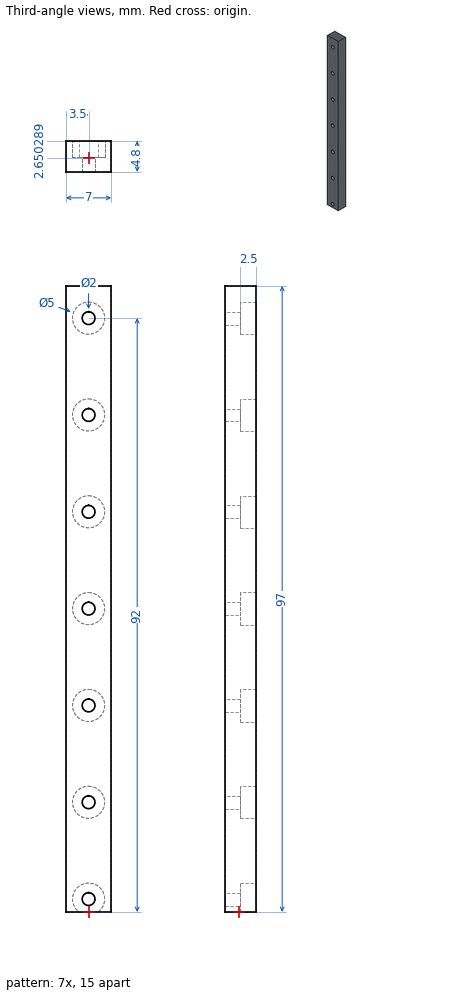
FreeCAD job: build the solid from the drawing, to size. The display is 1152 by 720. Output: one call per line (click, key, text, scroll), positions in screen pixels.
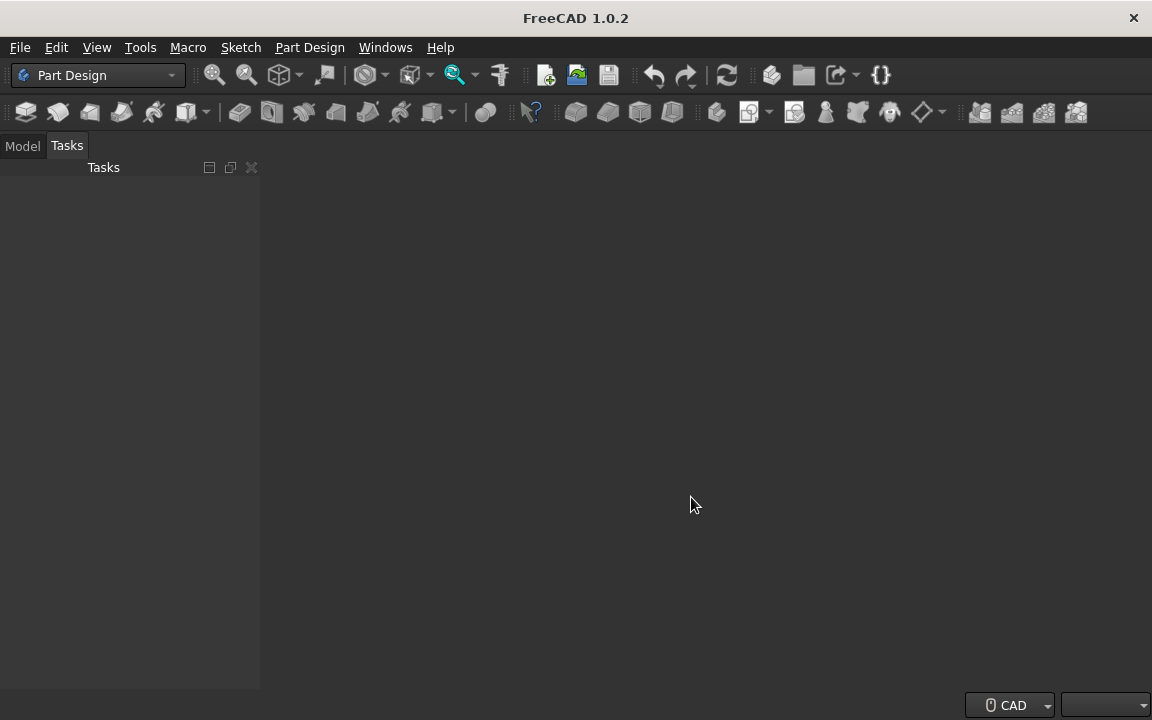
click(546, 76)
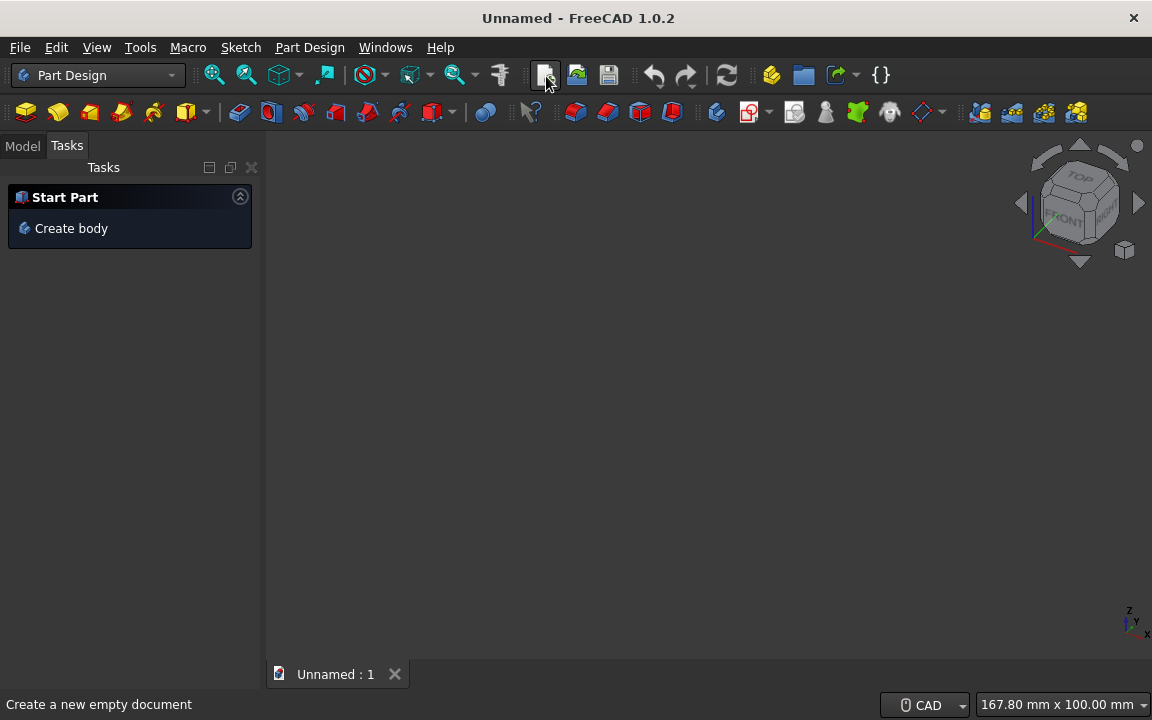
click(750, 112)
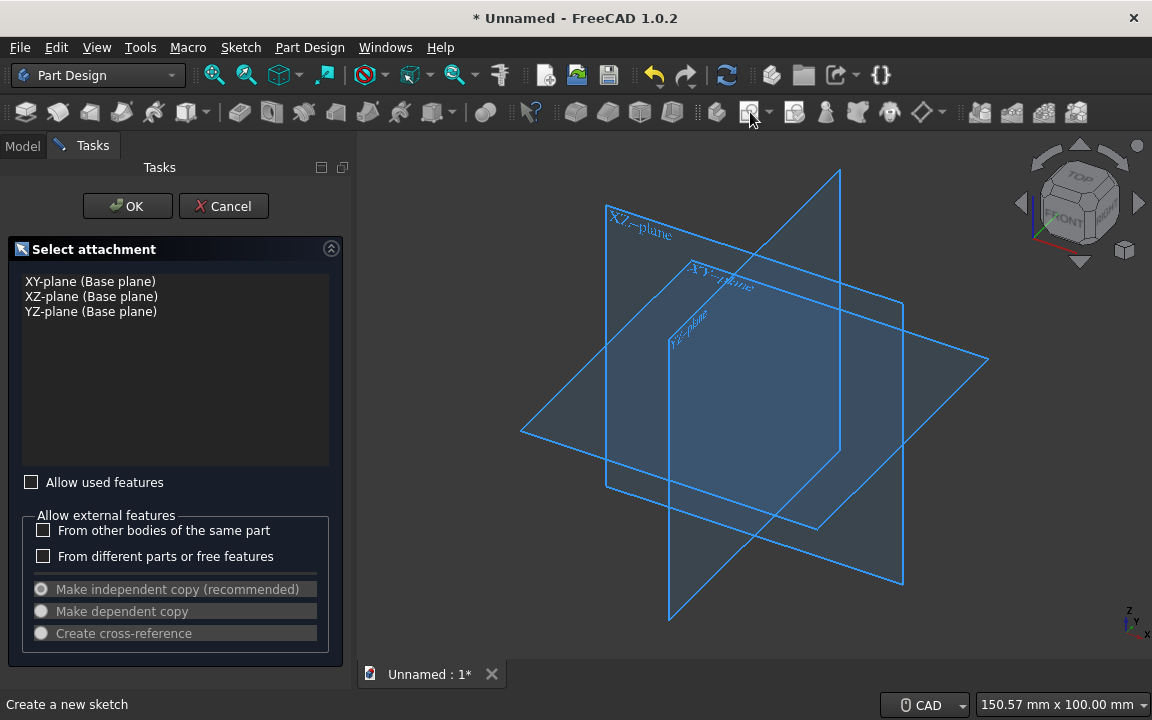
click(82, 282)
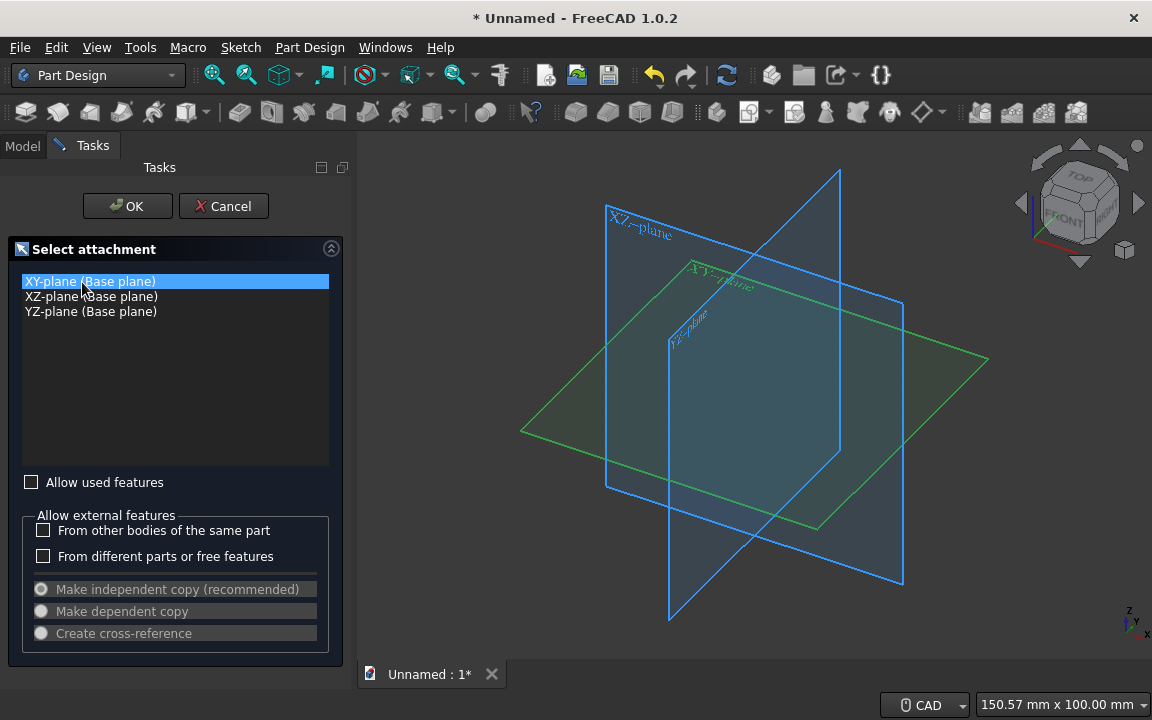
click(128, 206)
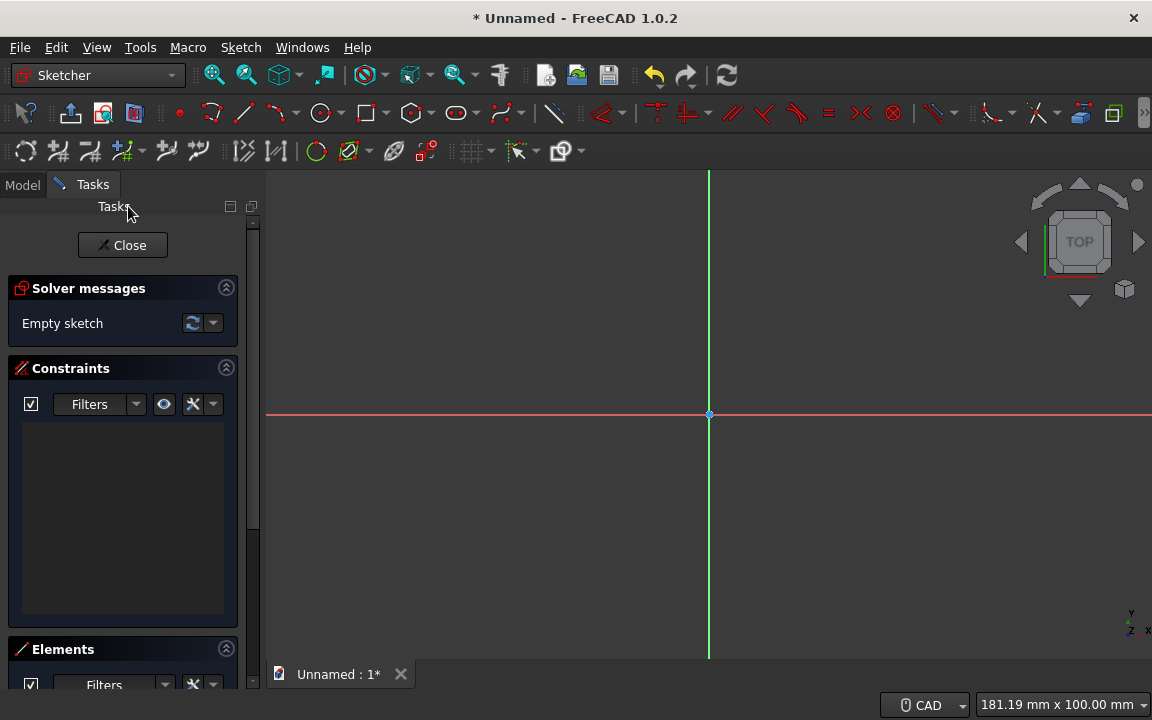
scroll(714, 413, up, 13)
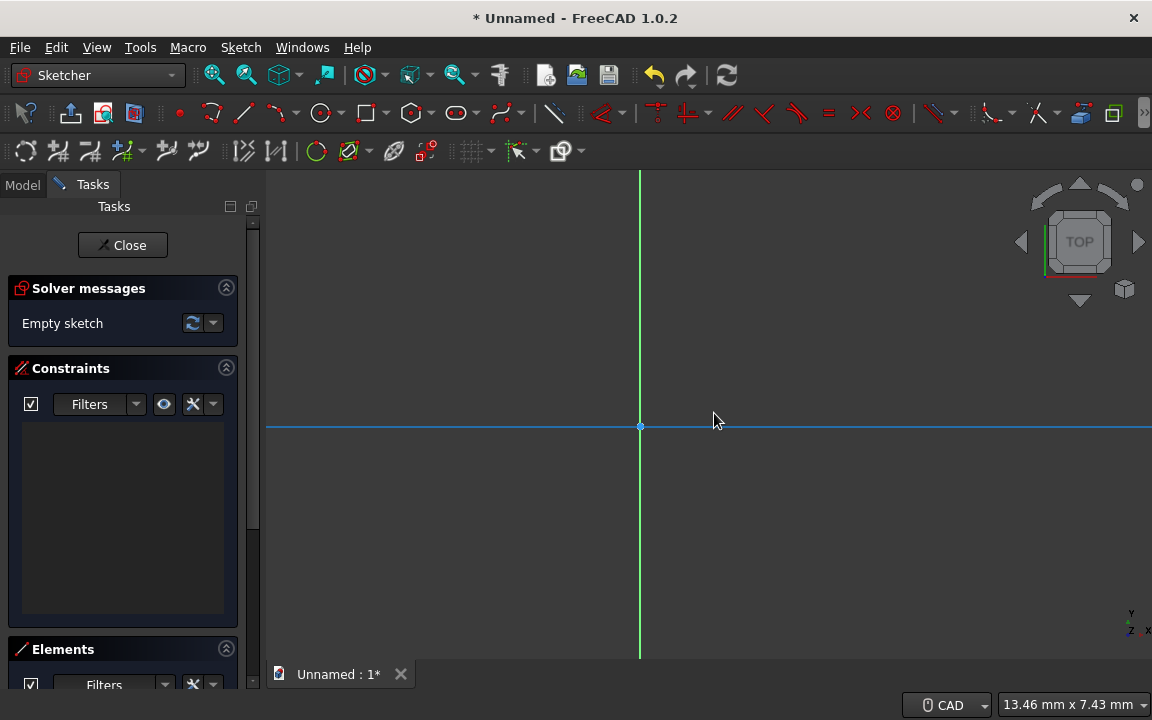
click(366, 114)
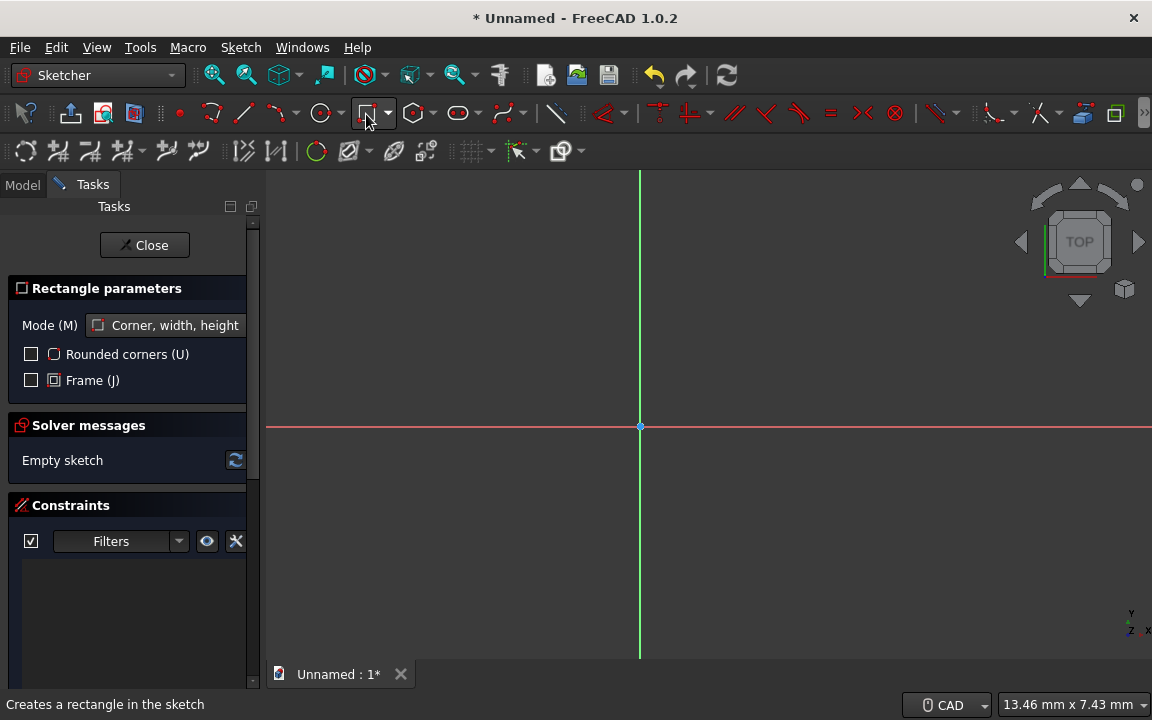
click(410, 253)
move(871, 569)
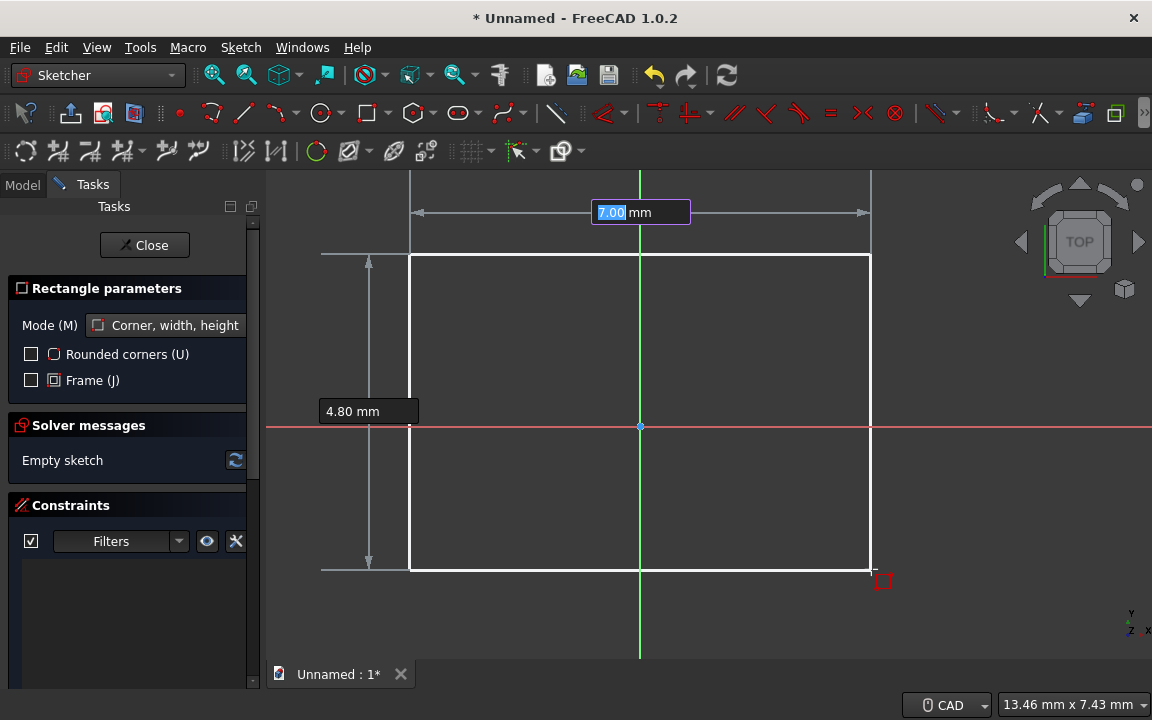
text(7)
key(Tab)
text(4.8)
key(Return)
key(Escape)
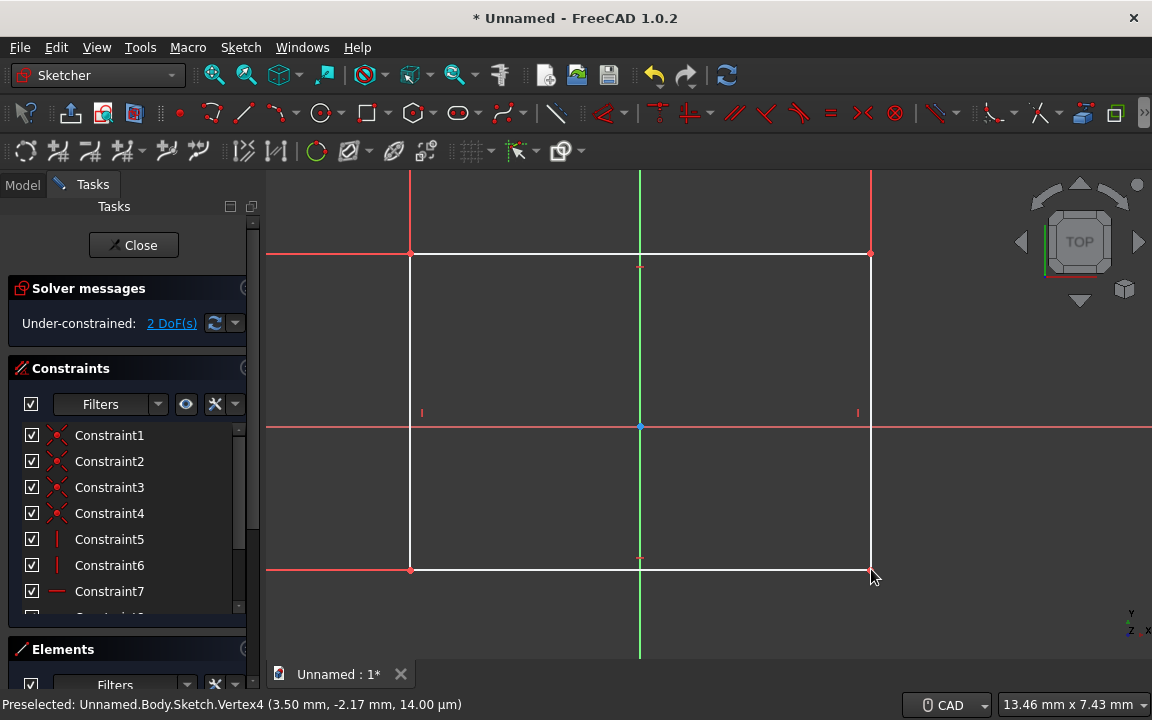
click(604, 114)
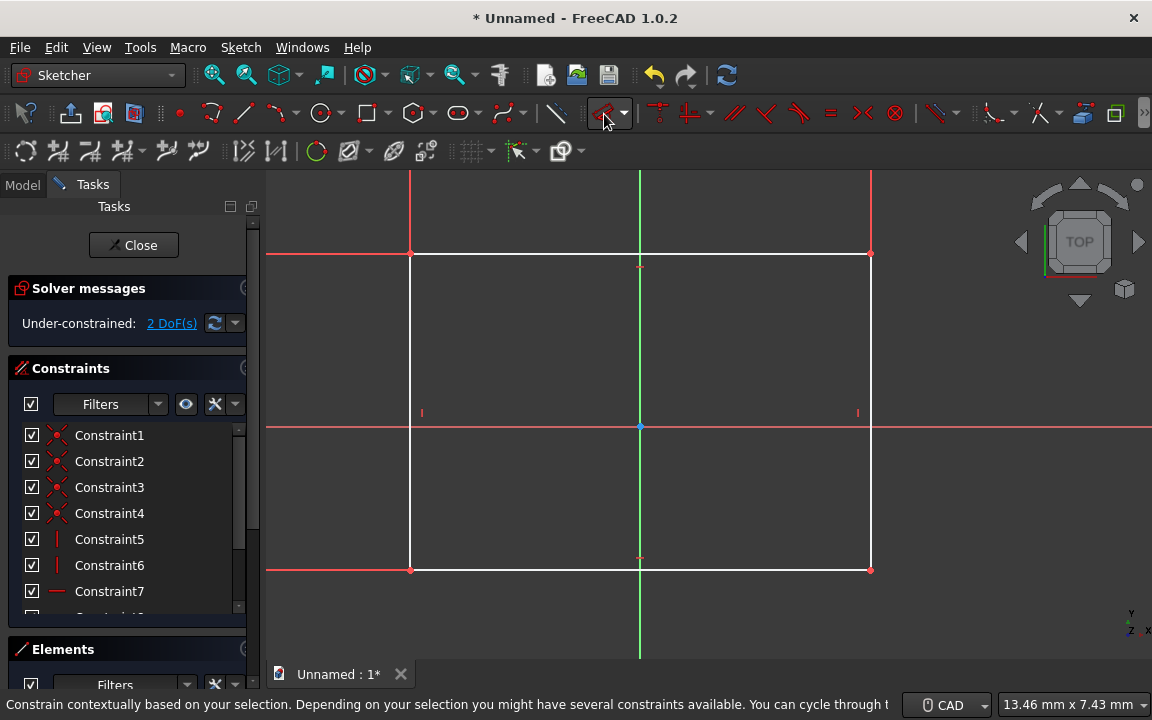
click(410, 254)
click(525, 220)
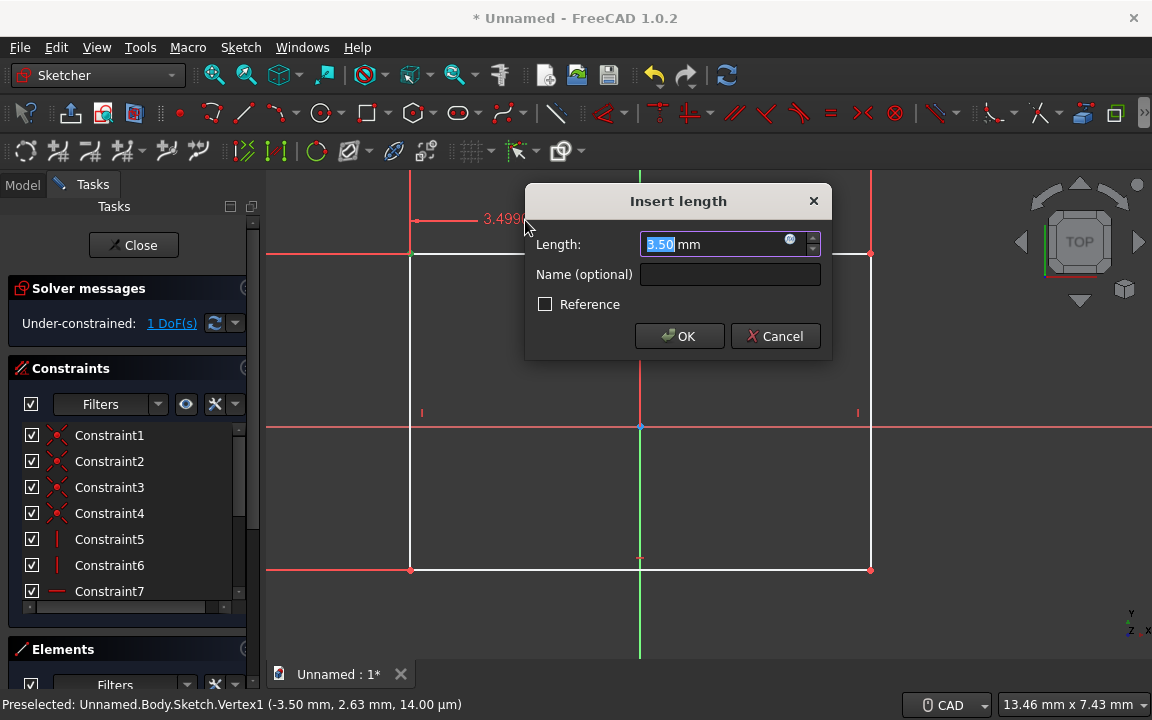
text(3.5)
key(Return)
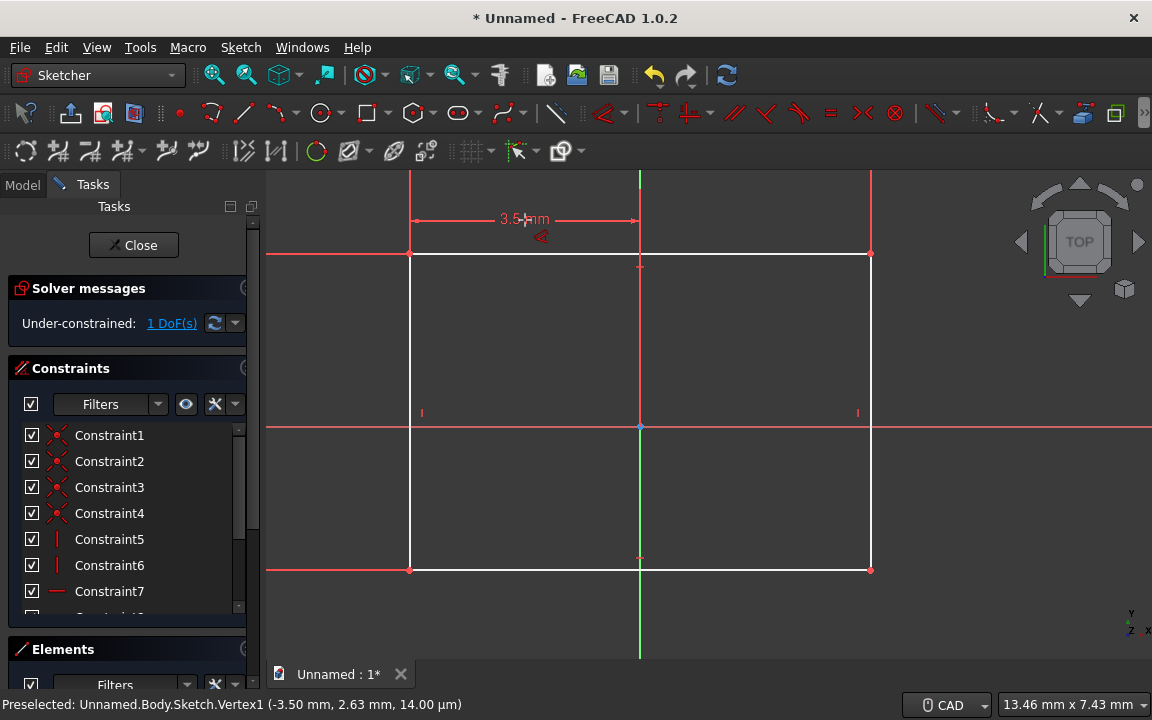
click(410, 254)
click(376, 340)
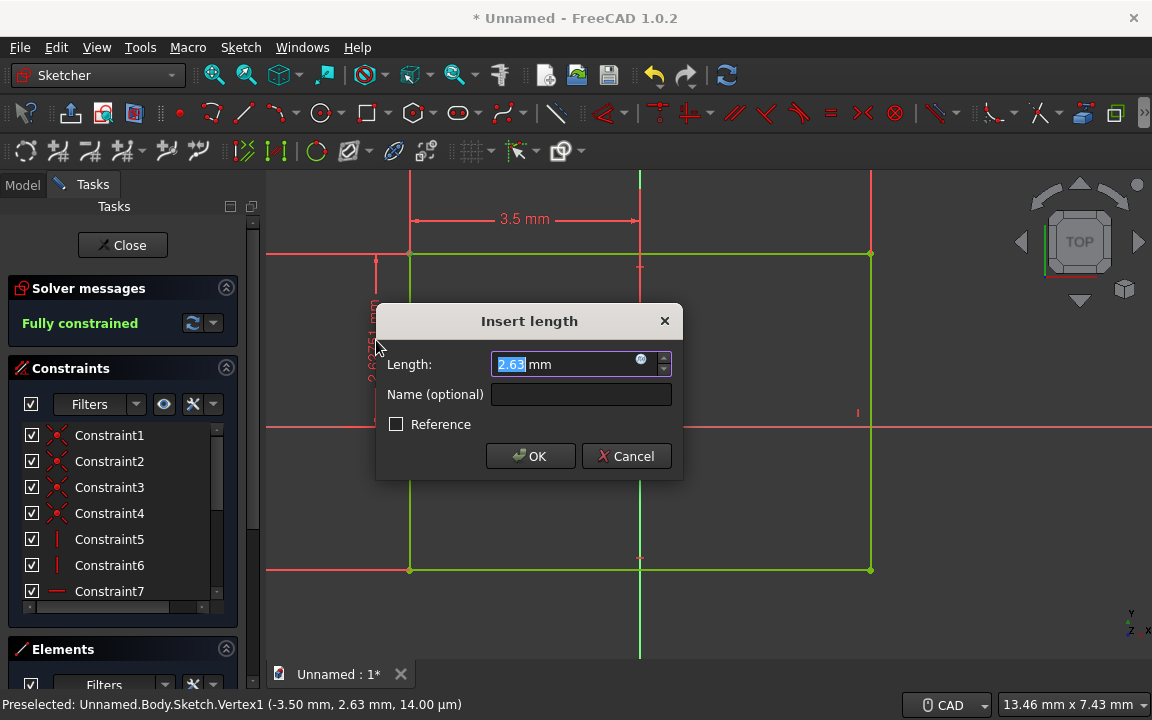
text(2.650289)
key(Return)
key(Escape)